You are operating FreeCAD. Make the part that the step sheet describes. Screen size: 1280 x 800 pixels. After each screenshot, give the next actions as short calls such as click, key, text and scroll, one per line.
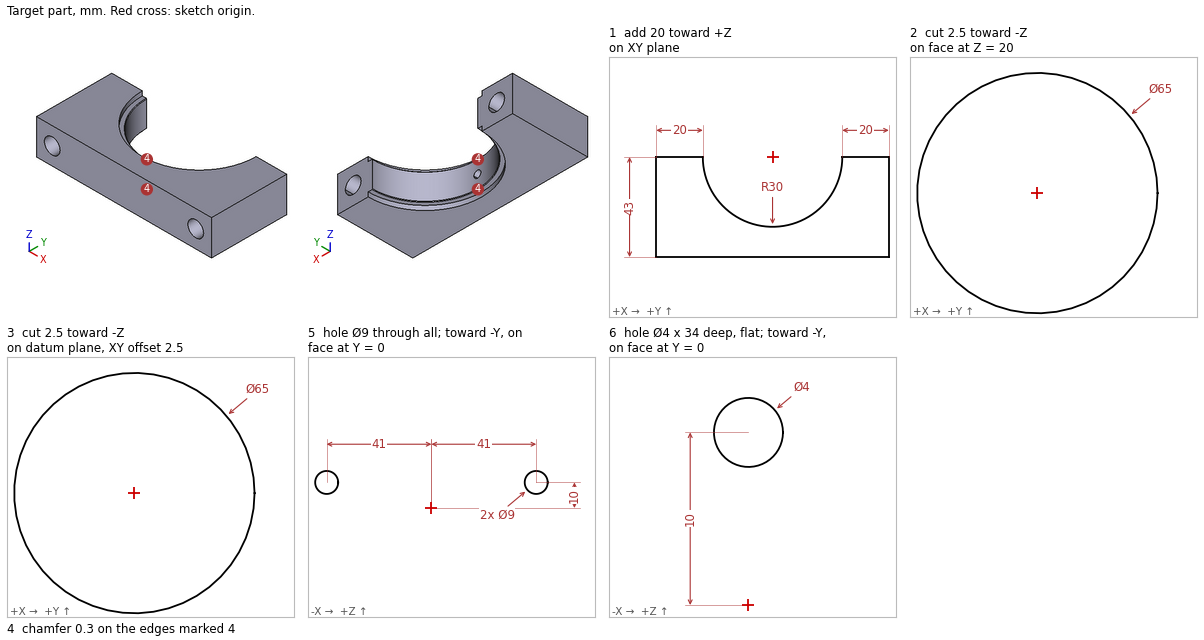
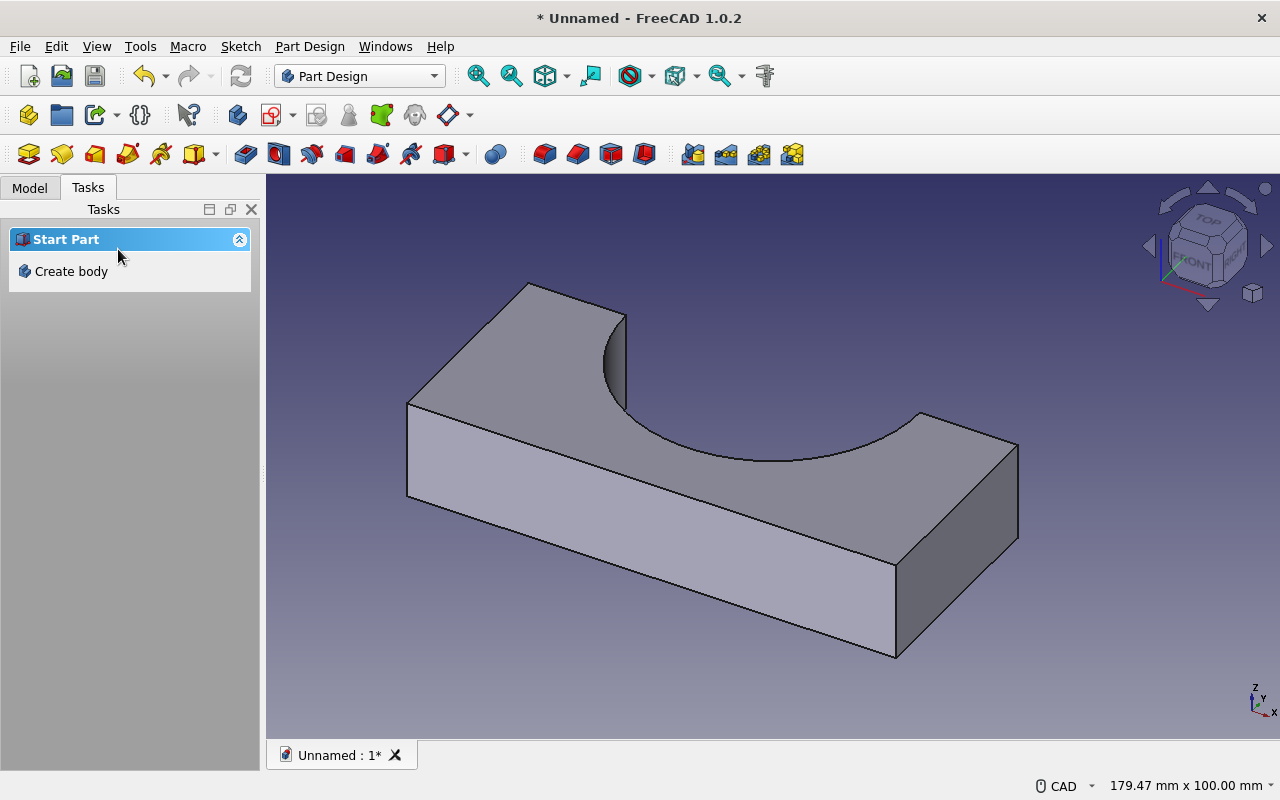
click(555, 394)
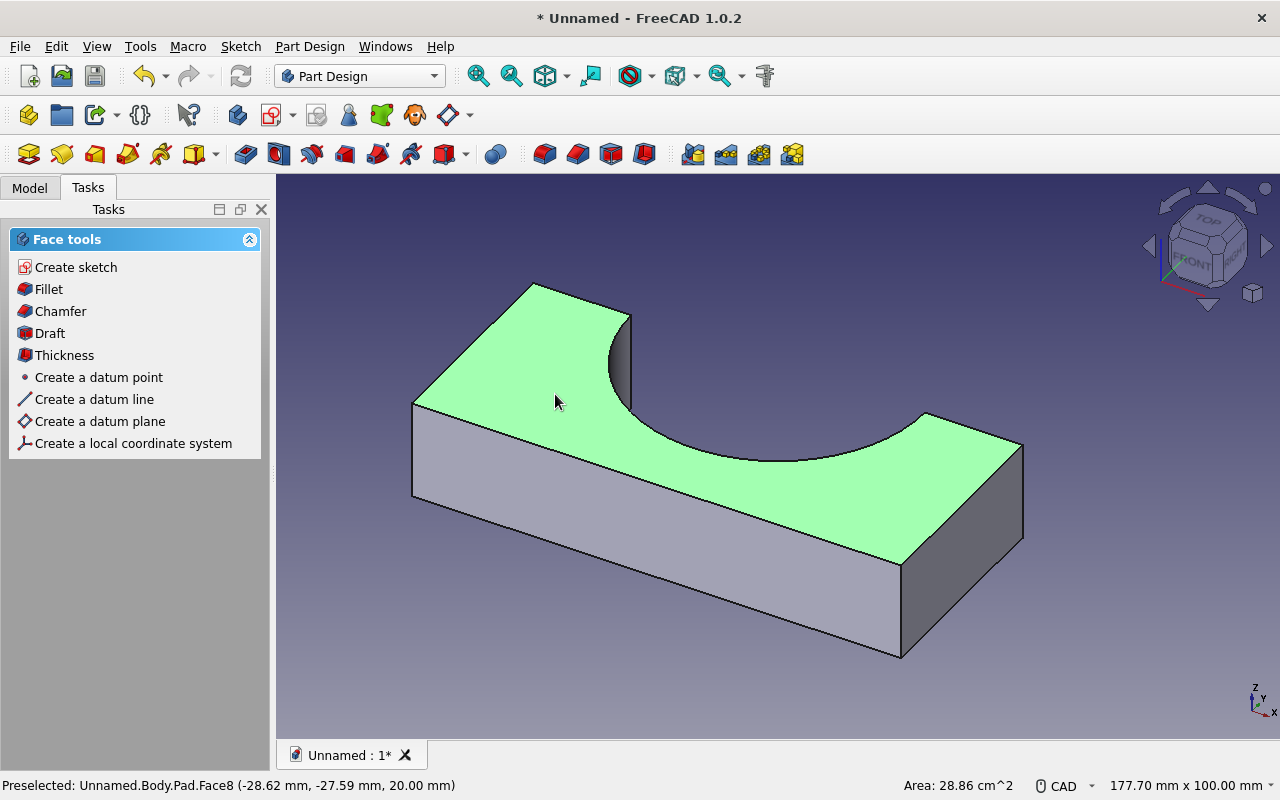
click(270, 116)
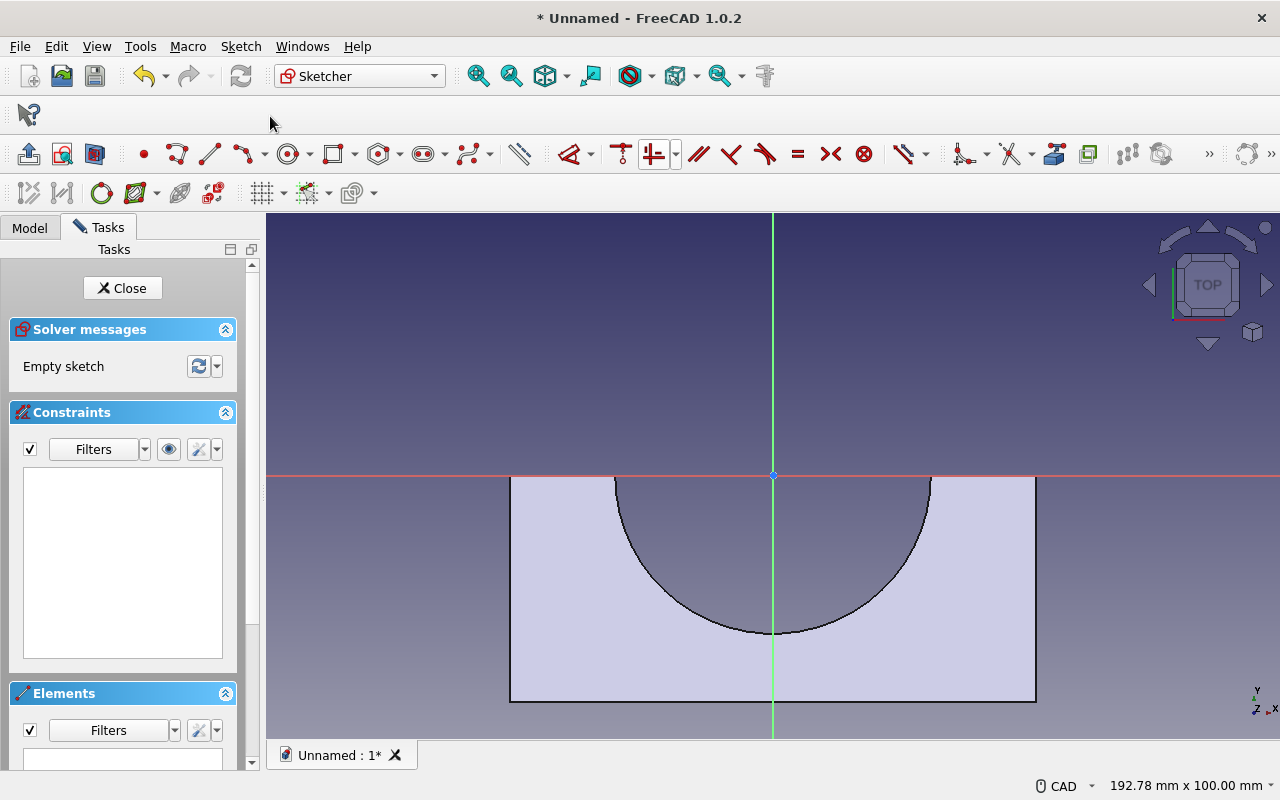
click(288, 154)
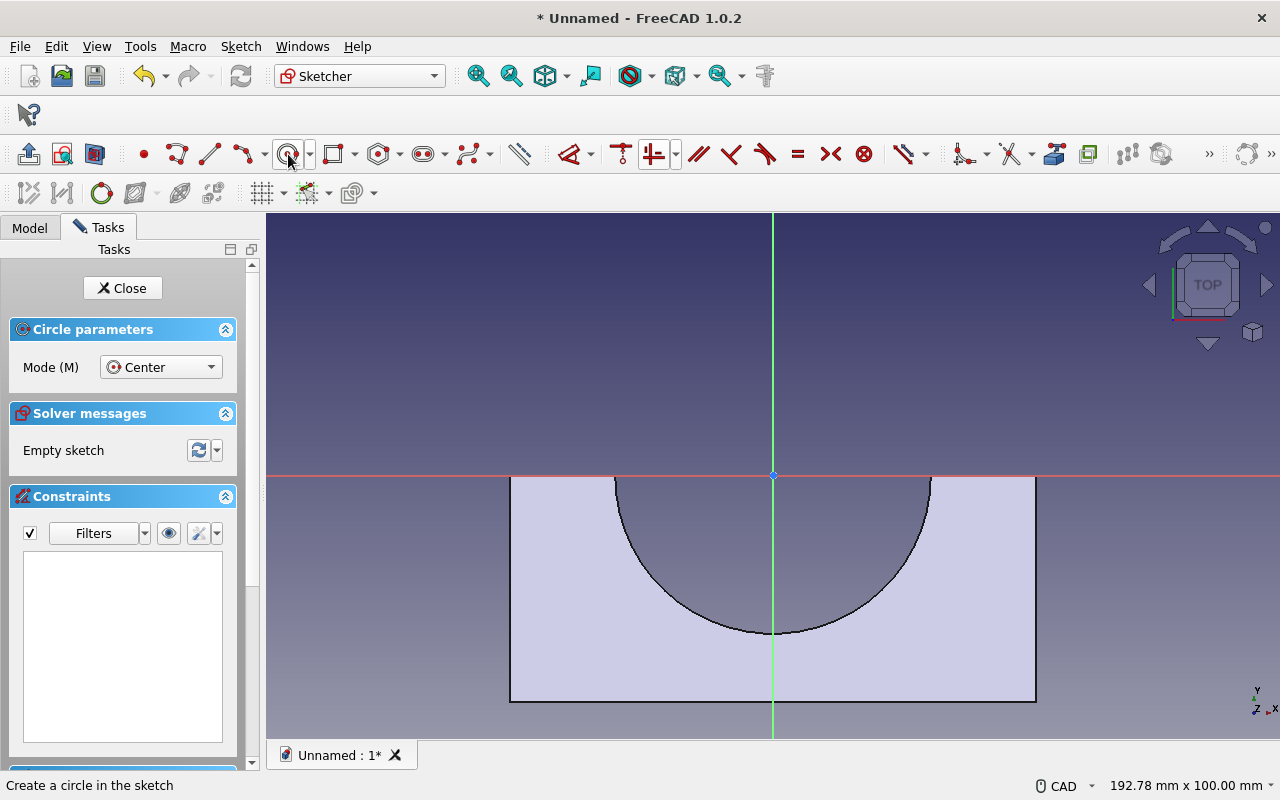
click(773, 476)
click(894, 355)
key(Escape)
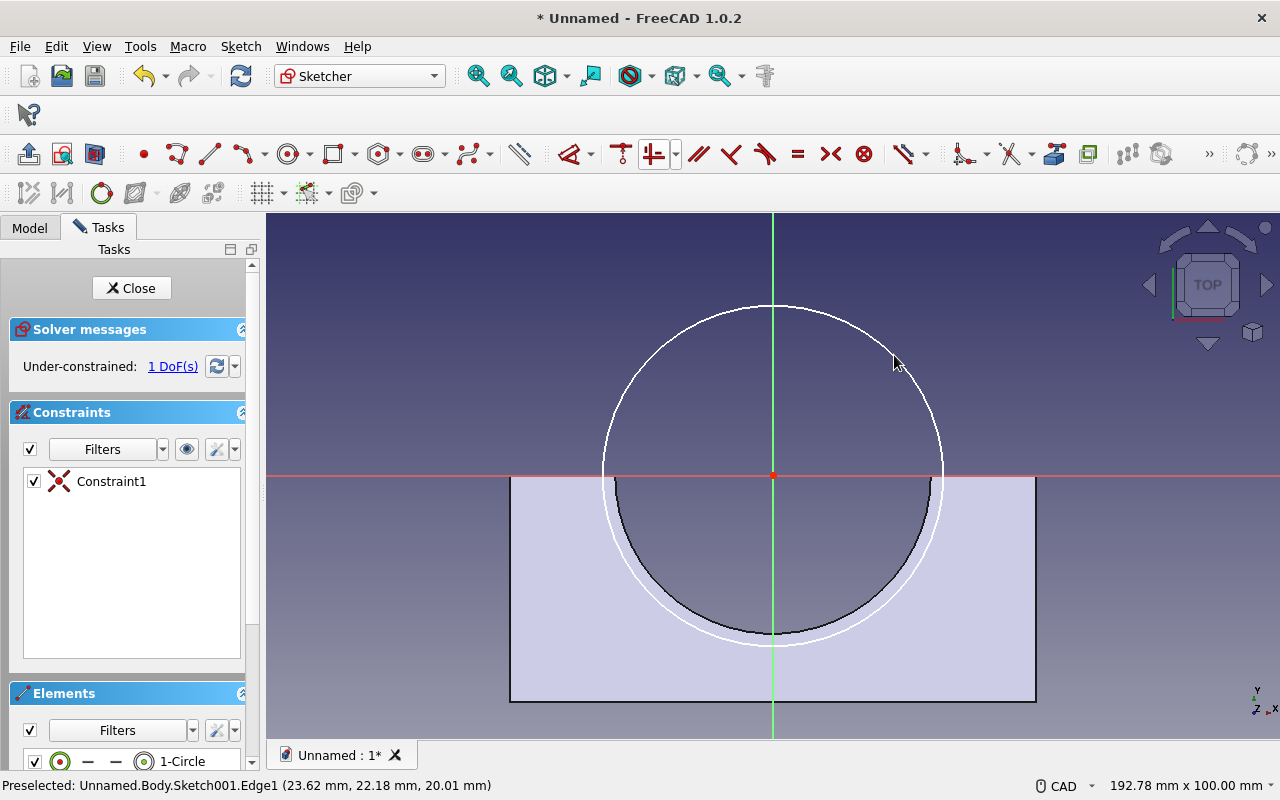
click(568, 154)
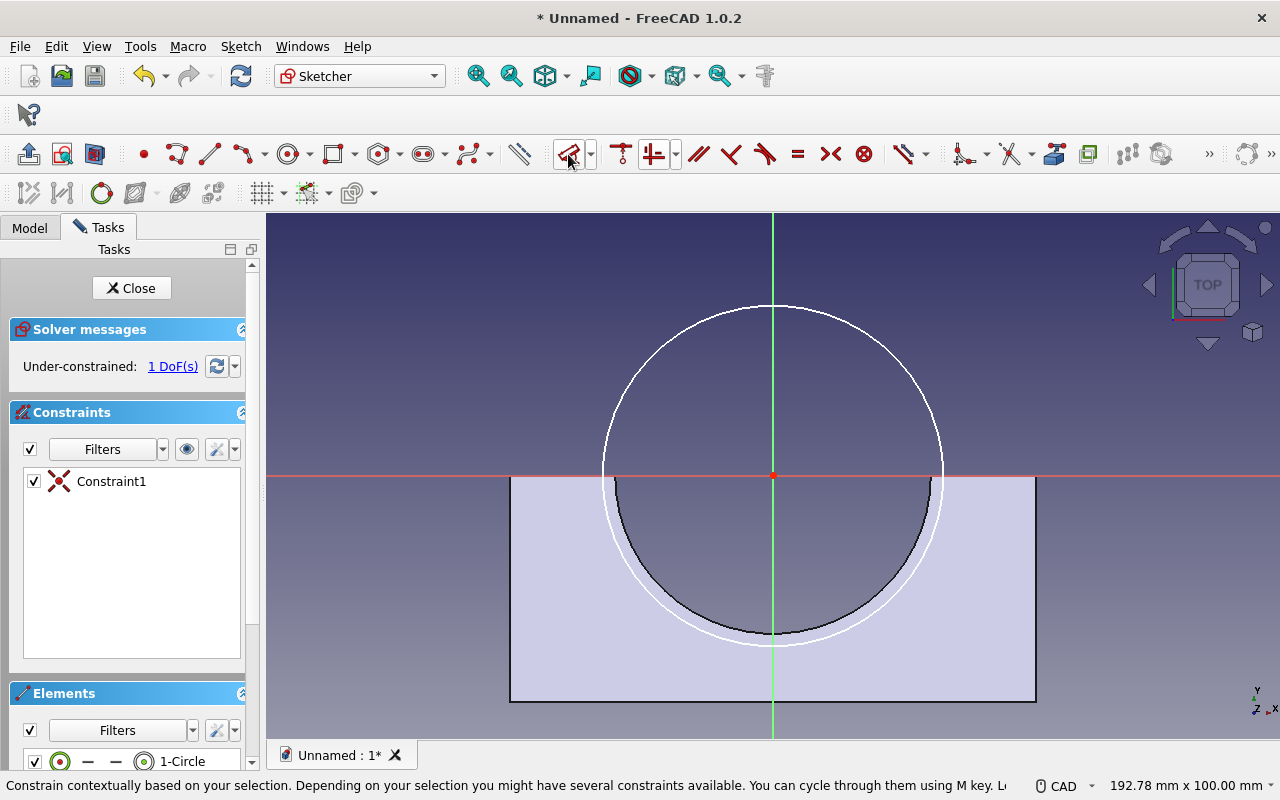
click(893, 355)
click(916, 332)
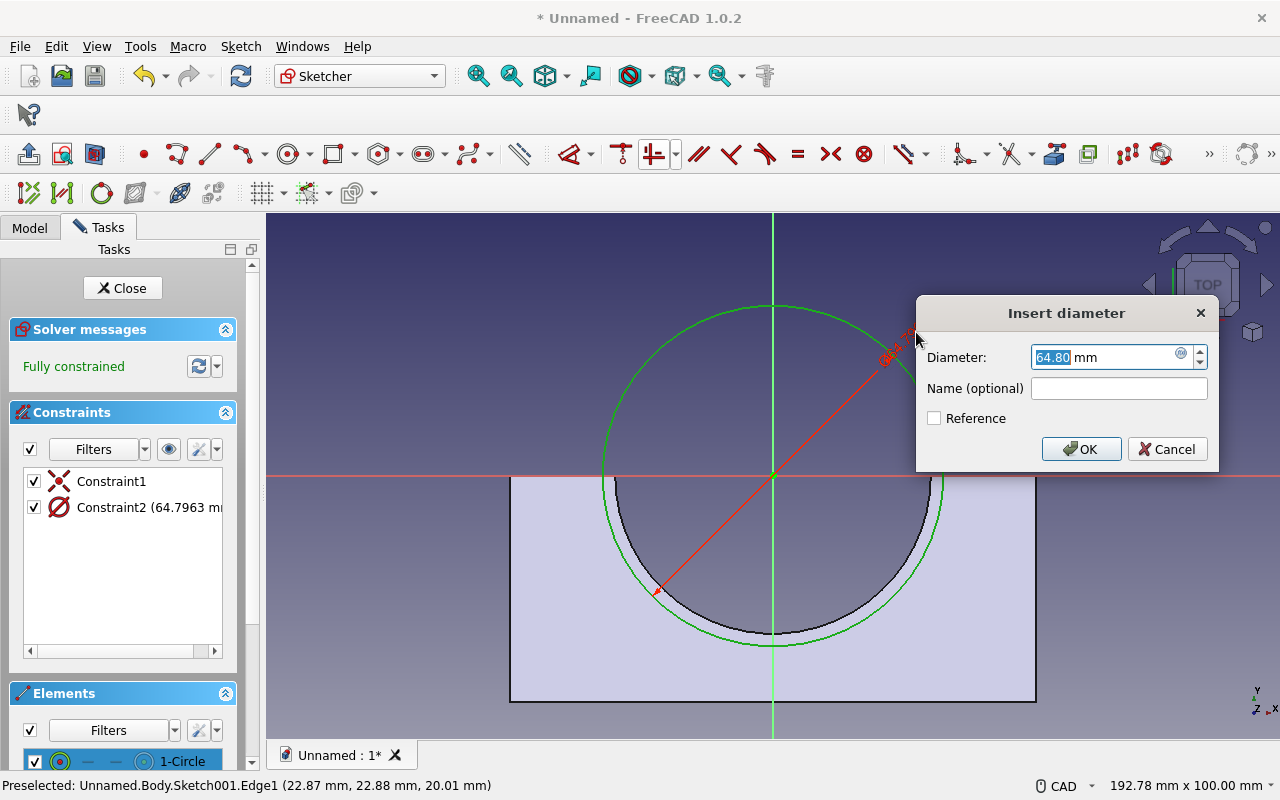
text(65)
key(Return)
key(Escape)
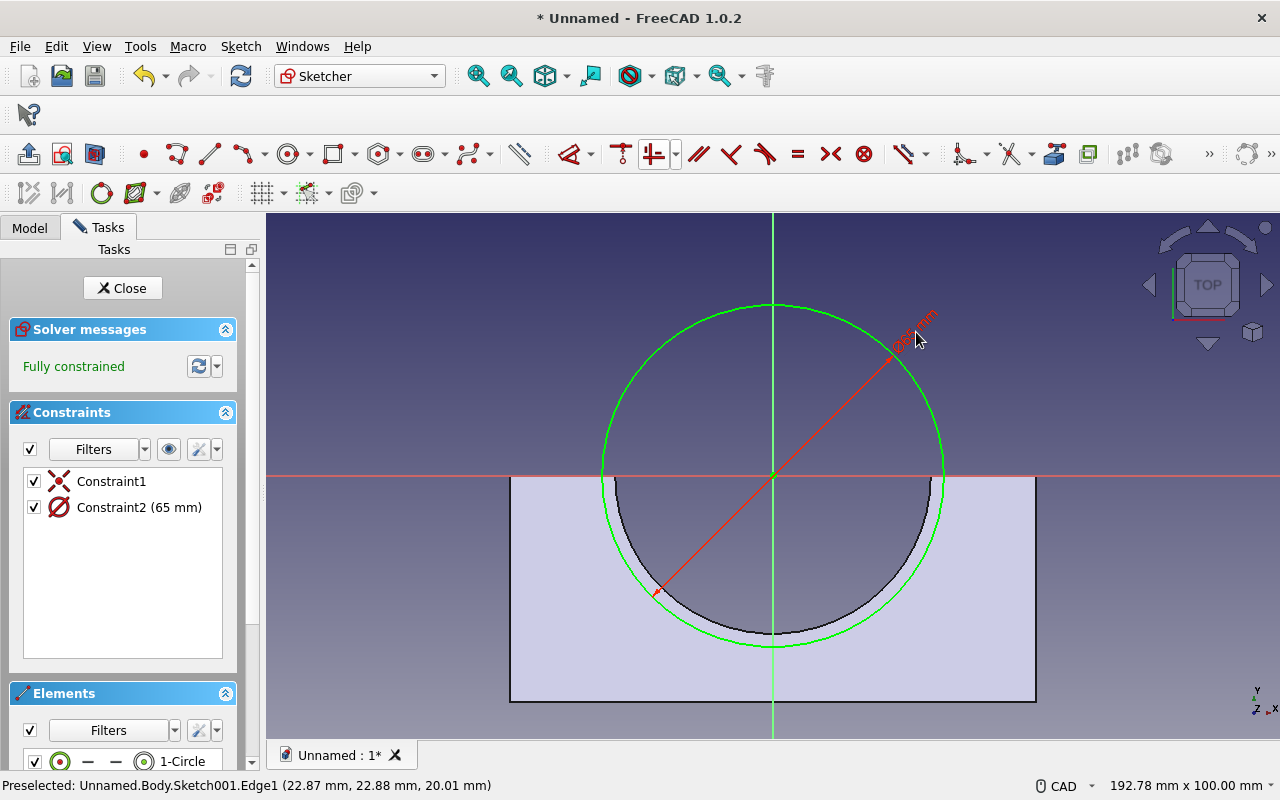
click(123, 288)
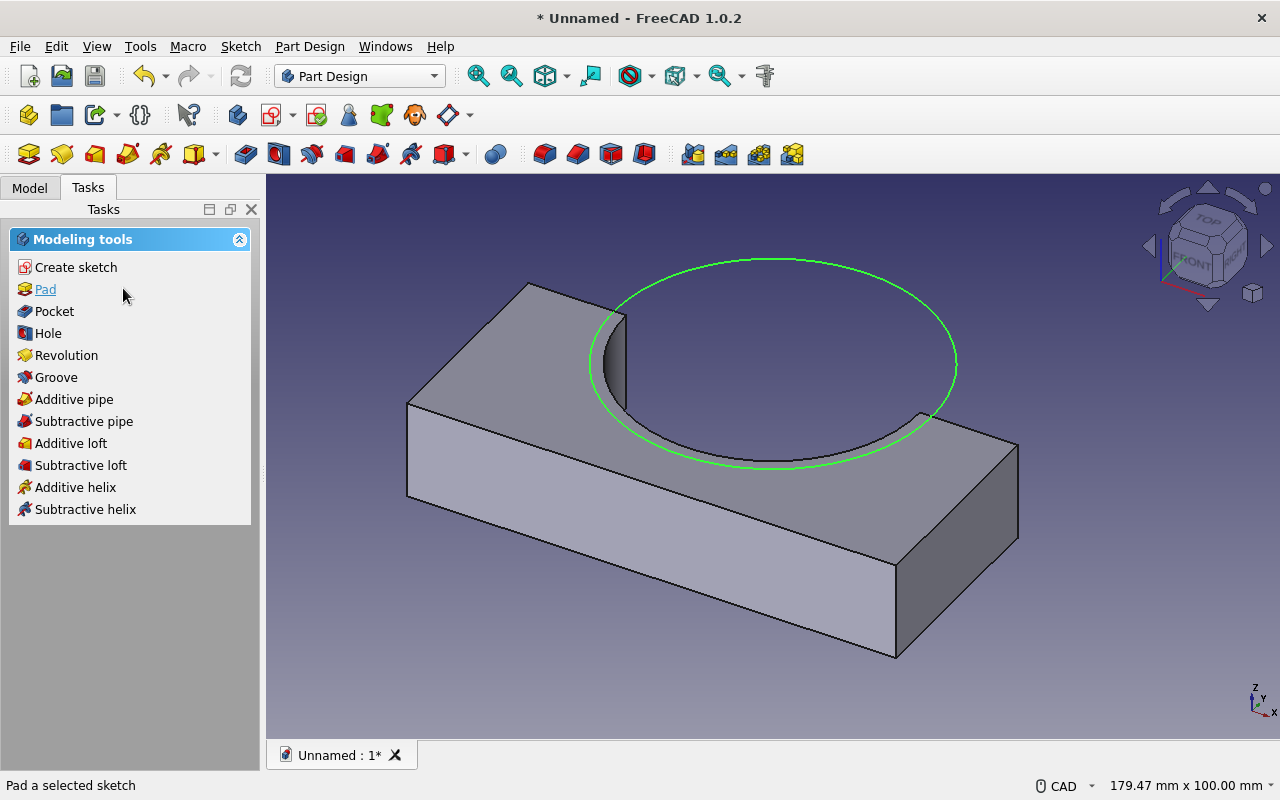
click(246, 154)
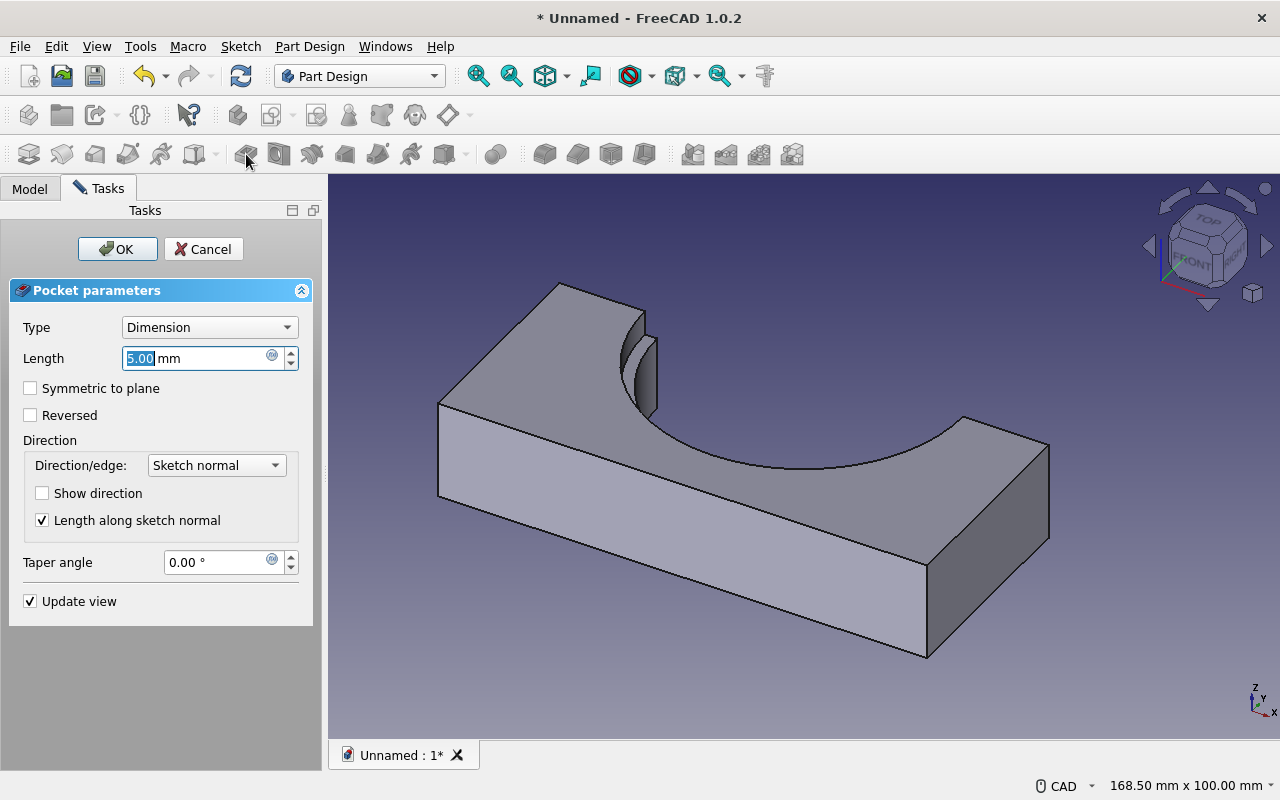
text(2.5)
key(Tab)